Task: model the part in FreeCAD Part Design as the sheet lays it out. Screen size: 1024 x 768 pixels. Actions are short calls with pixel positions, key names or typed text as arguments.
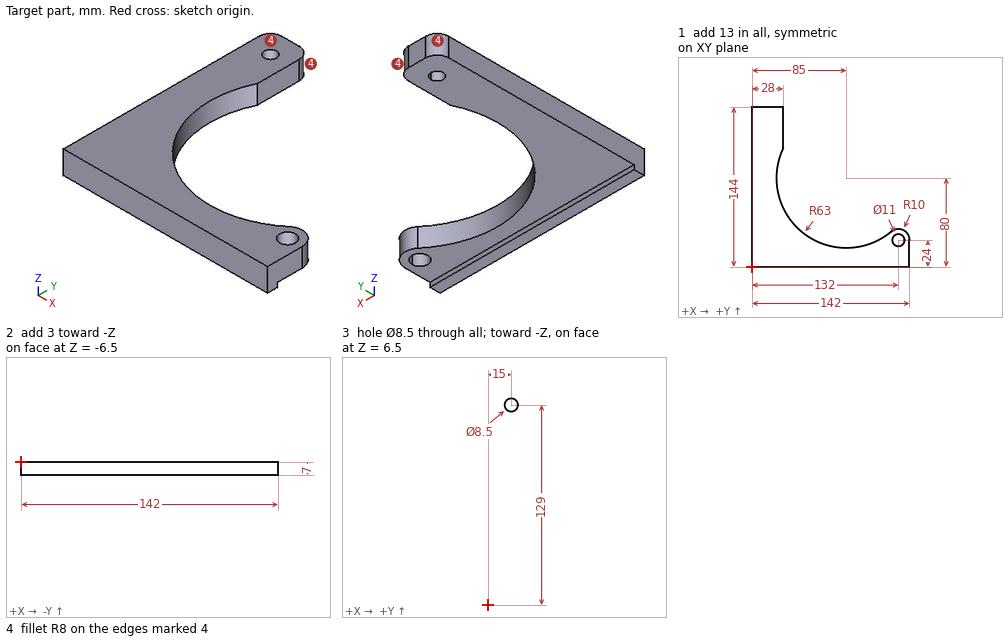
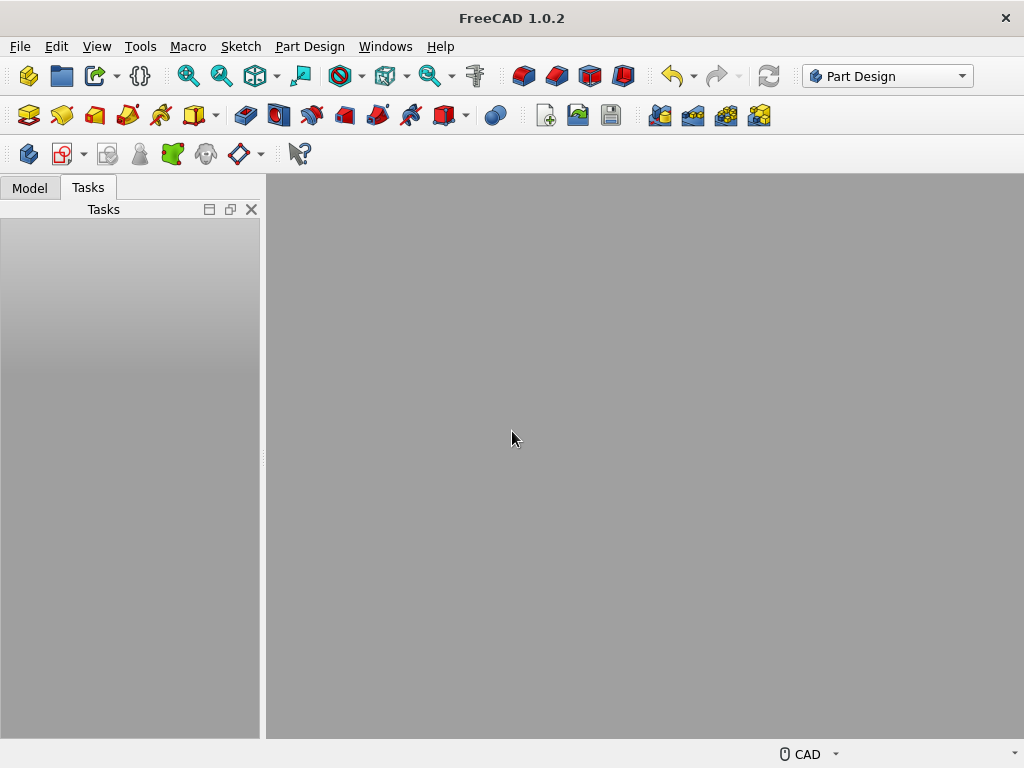
click(545, 116)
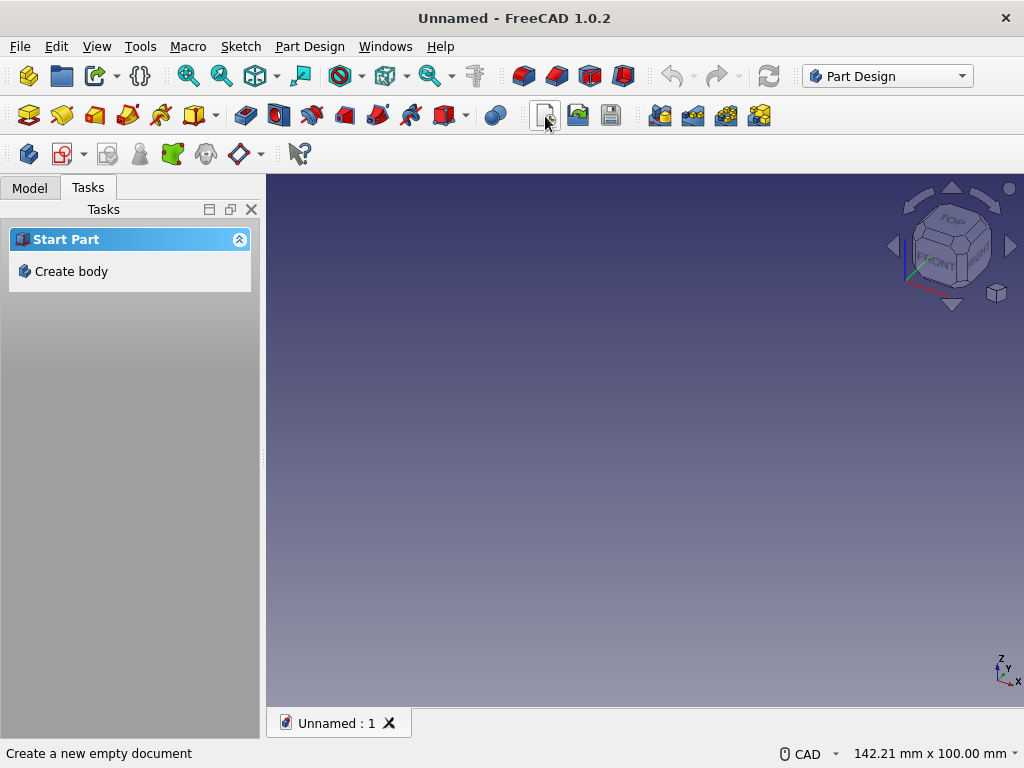
click(62, 154)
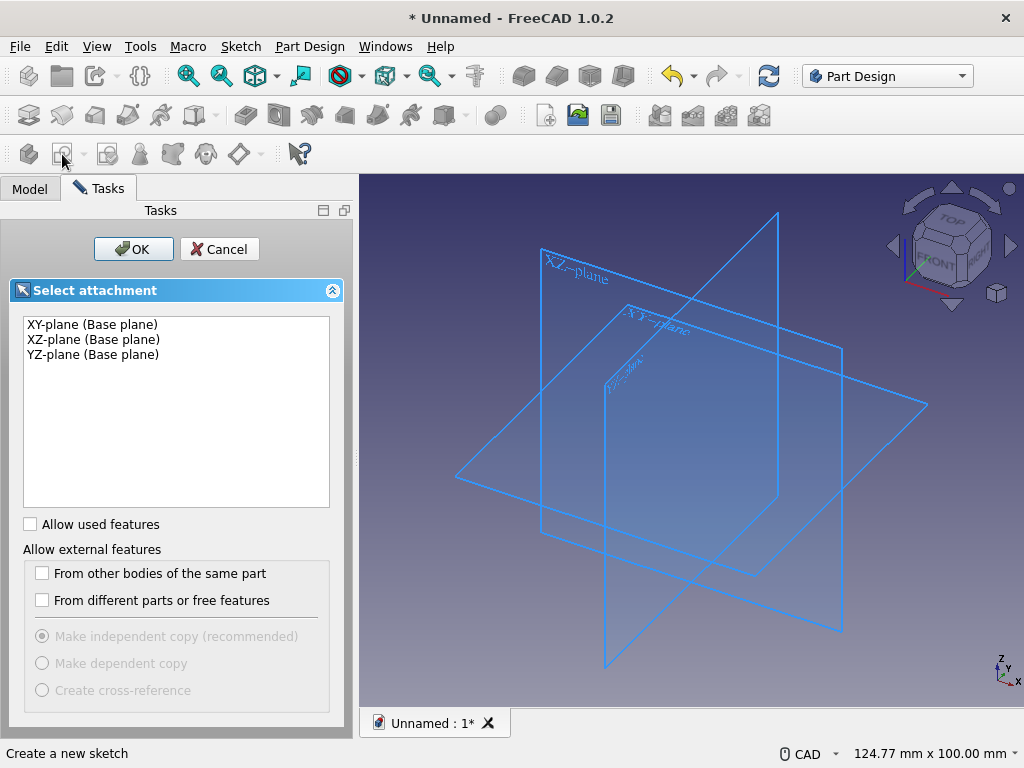
click(84, 324)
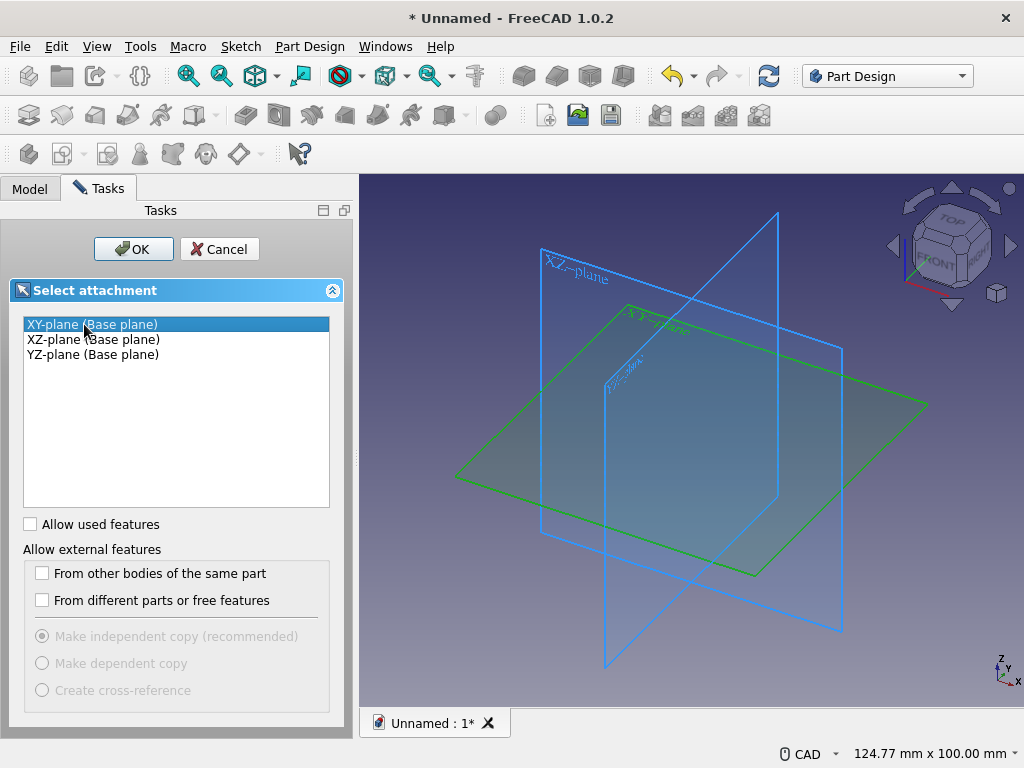
click(134, 249)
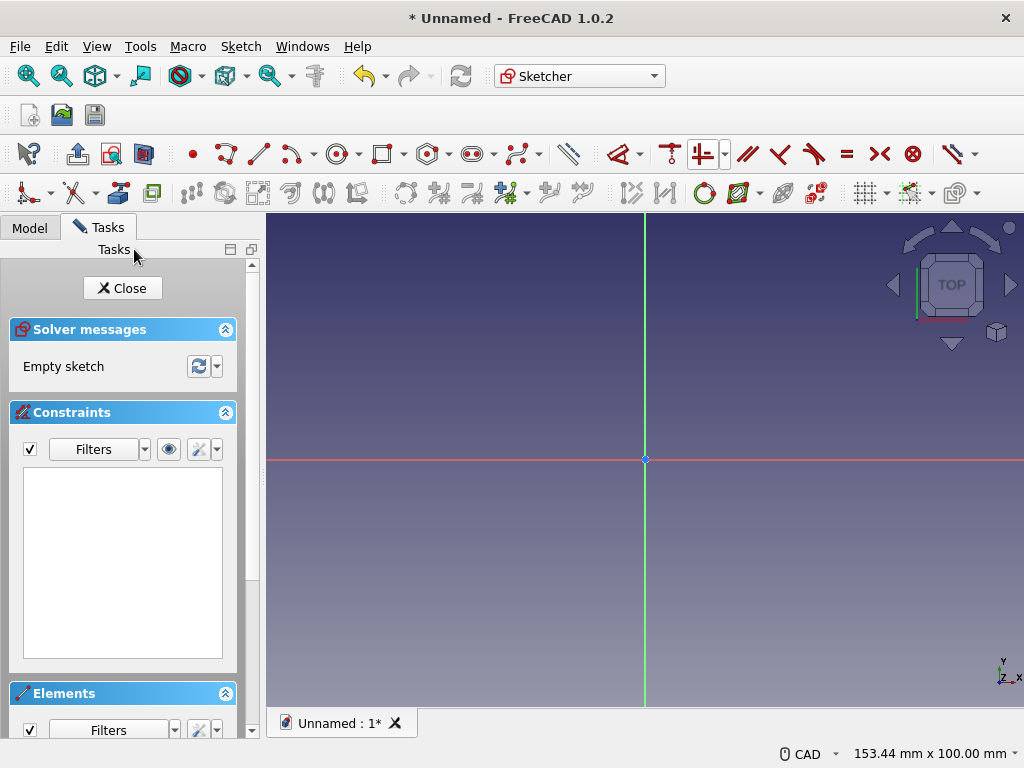
scroll(333, 667, down, 5)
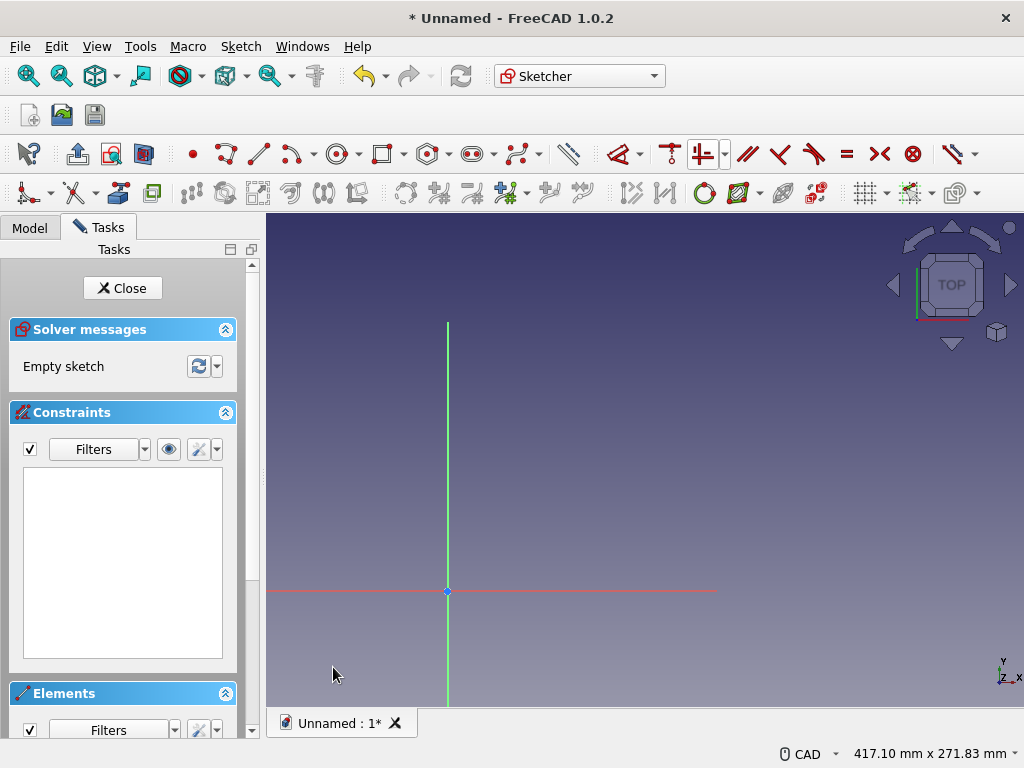
click(226, 154)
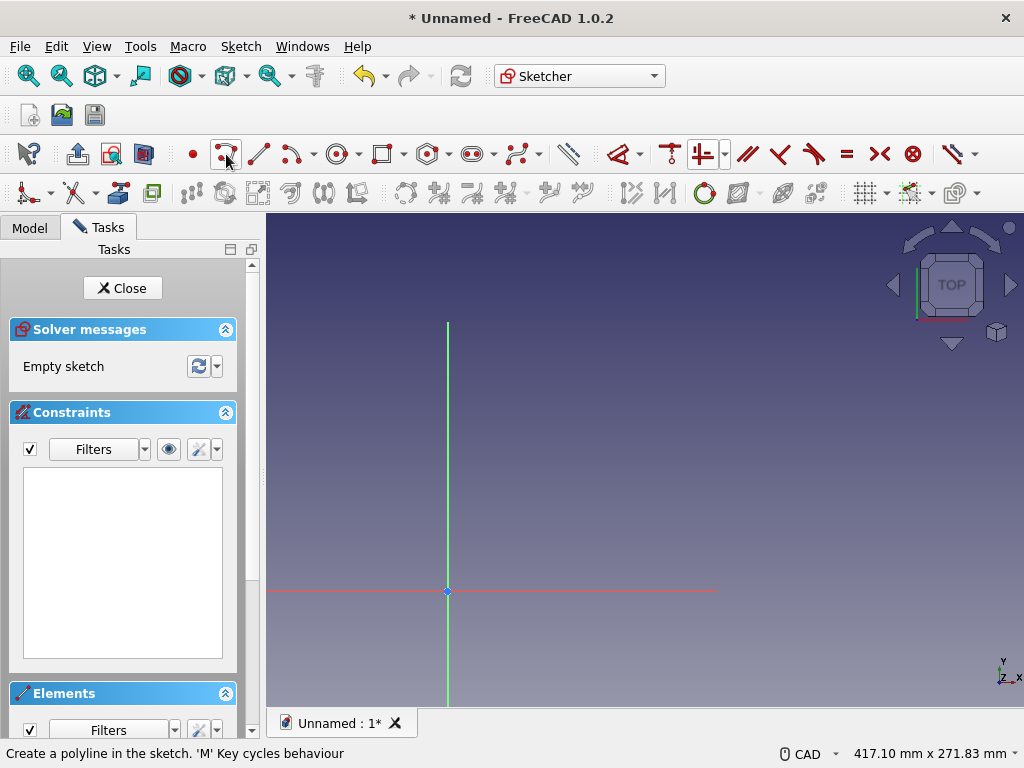
click(499, 397)
click(499, 330)
click(448, 330)
click(448, 591)
click(706, 582)
click(706, 548)
right_click(706, 548)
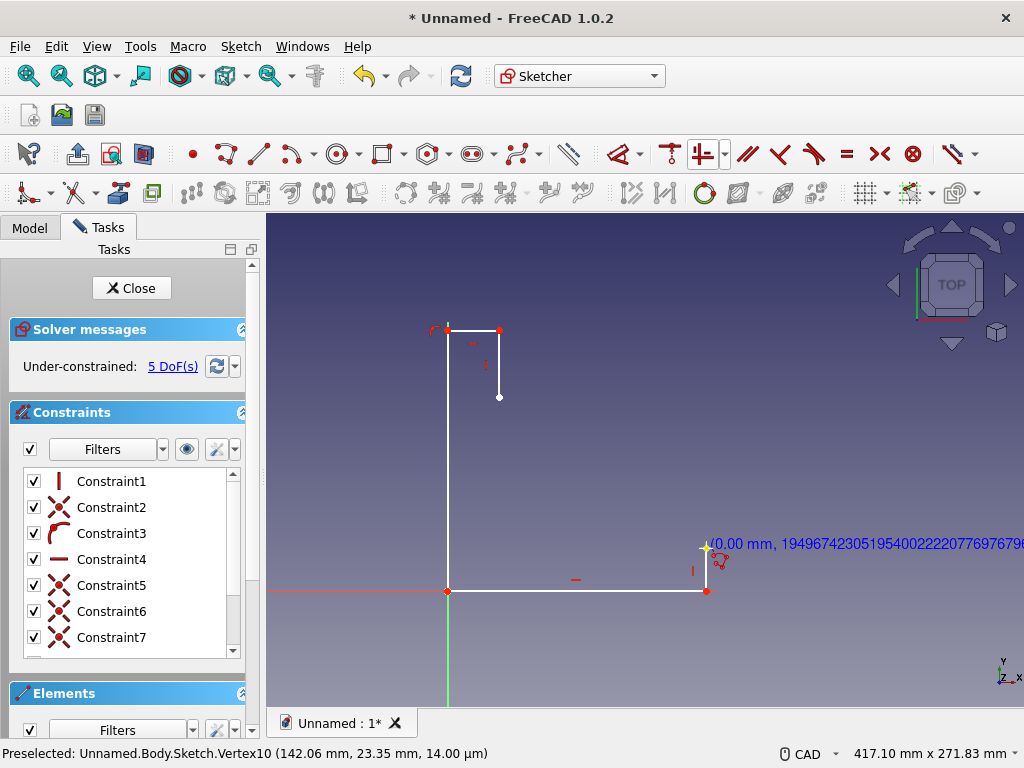
click(314, 154)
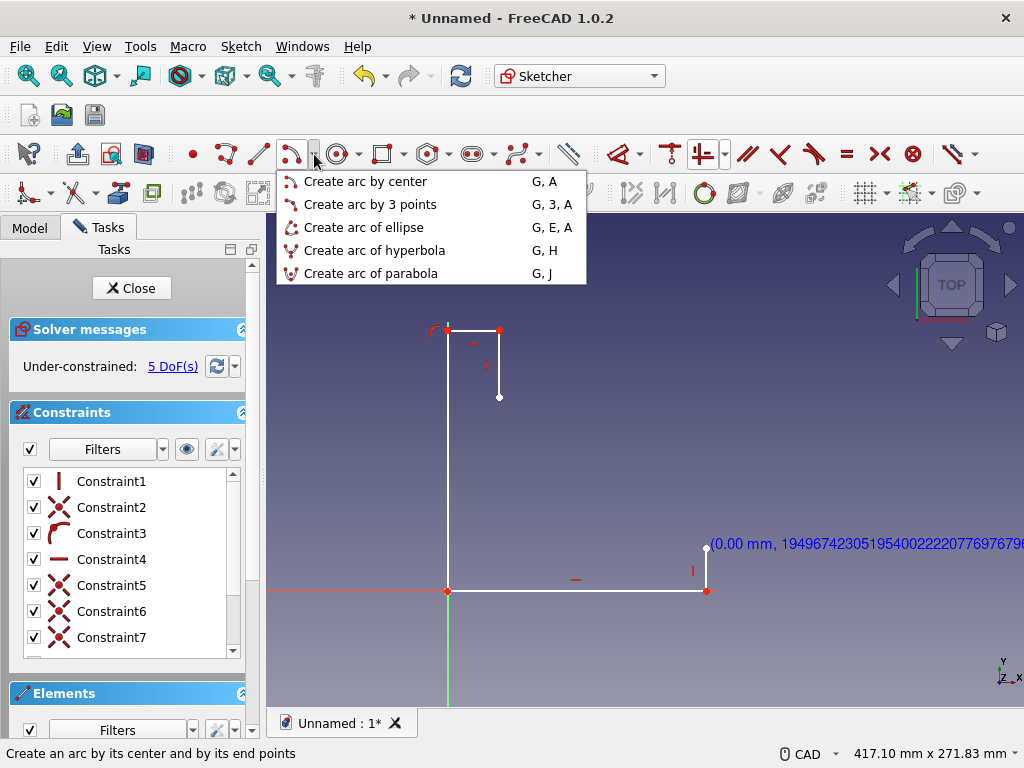
click(432, 204)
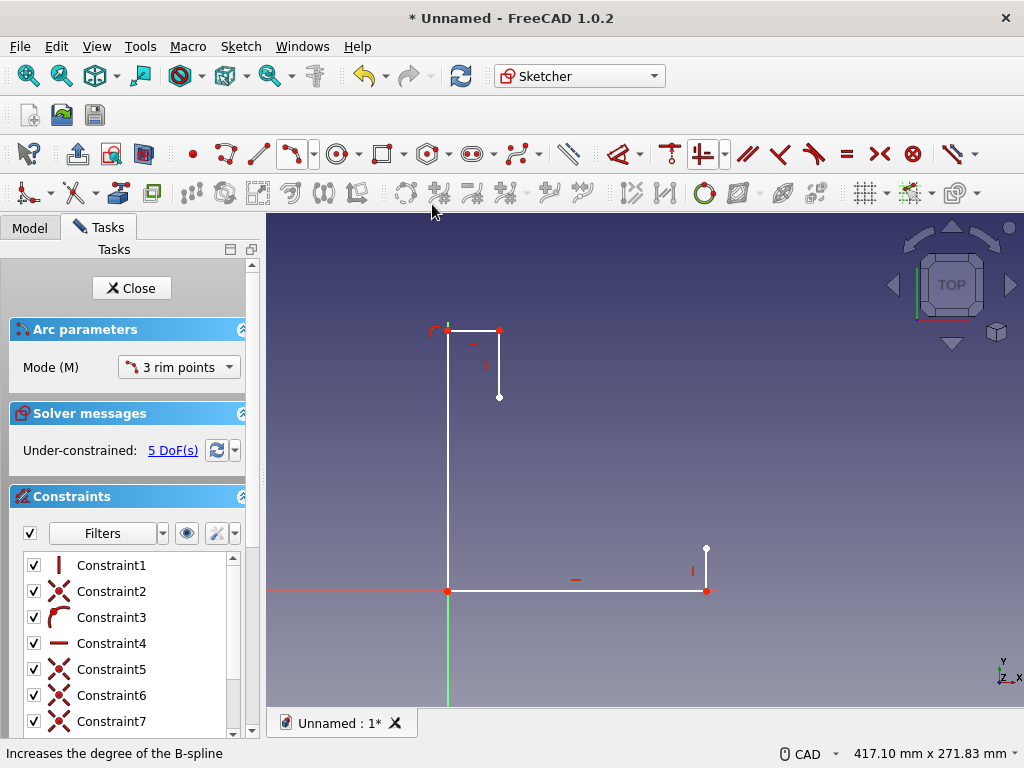
click(706, 549)
click(676, 534)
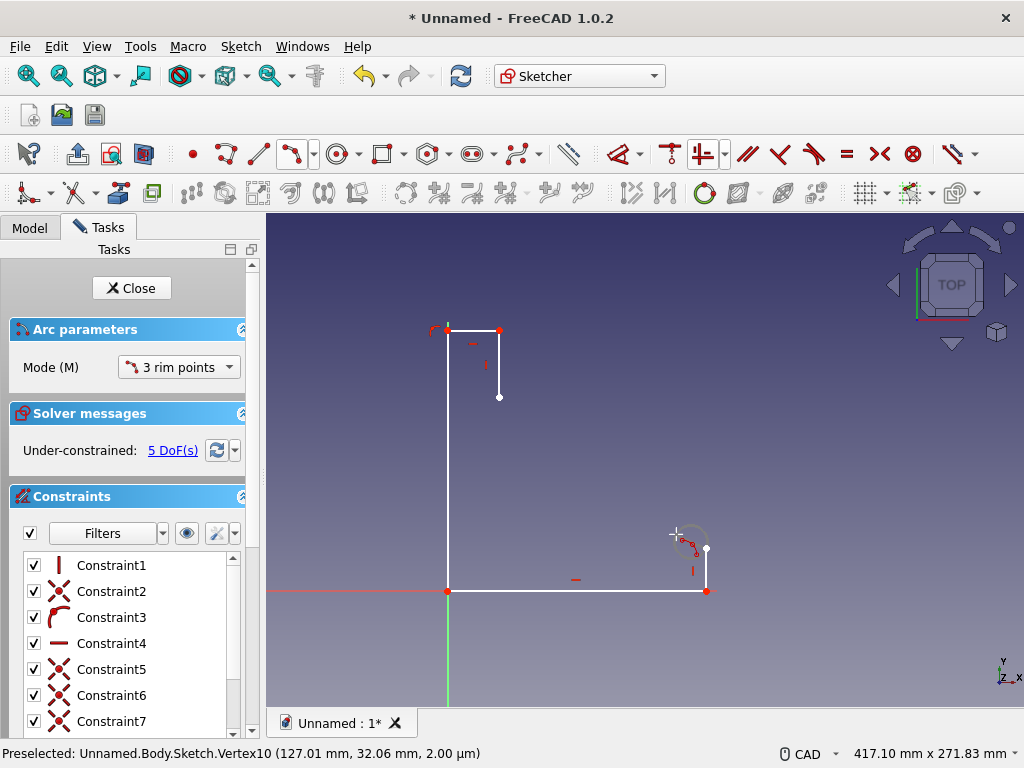
scroll(695, 531, up, 3)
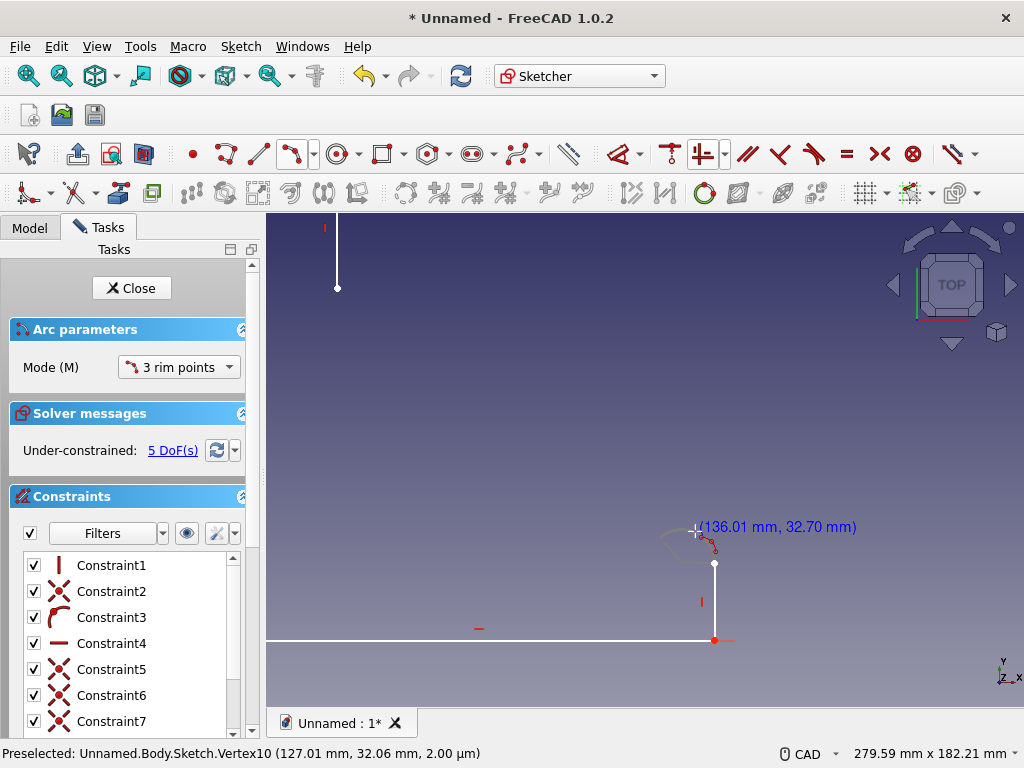
click(695, 531)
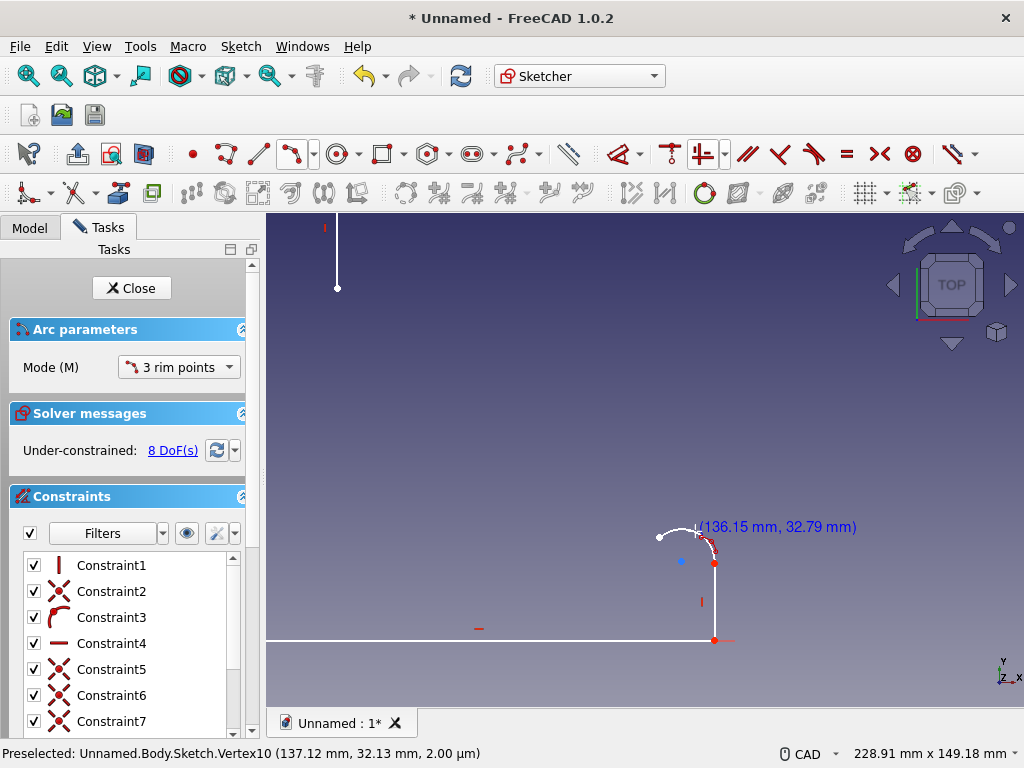
click(660, 538)
click(337, 288)
click(398, 541)